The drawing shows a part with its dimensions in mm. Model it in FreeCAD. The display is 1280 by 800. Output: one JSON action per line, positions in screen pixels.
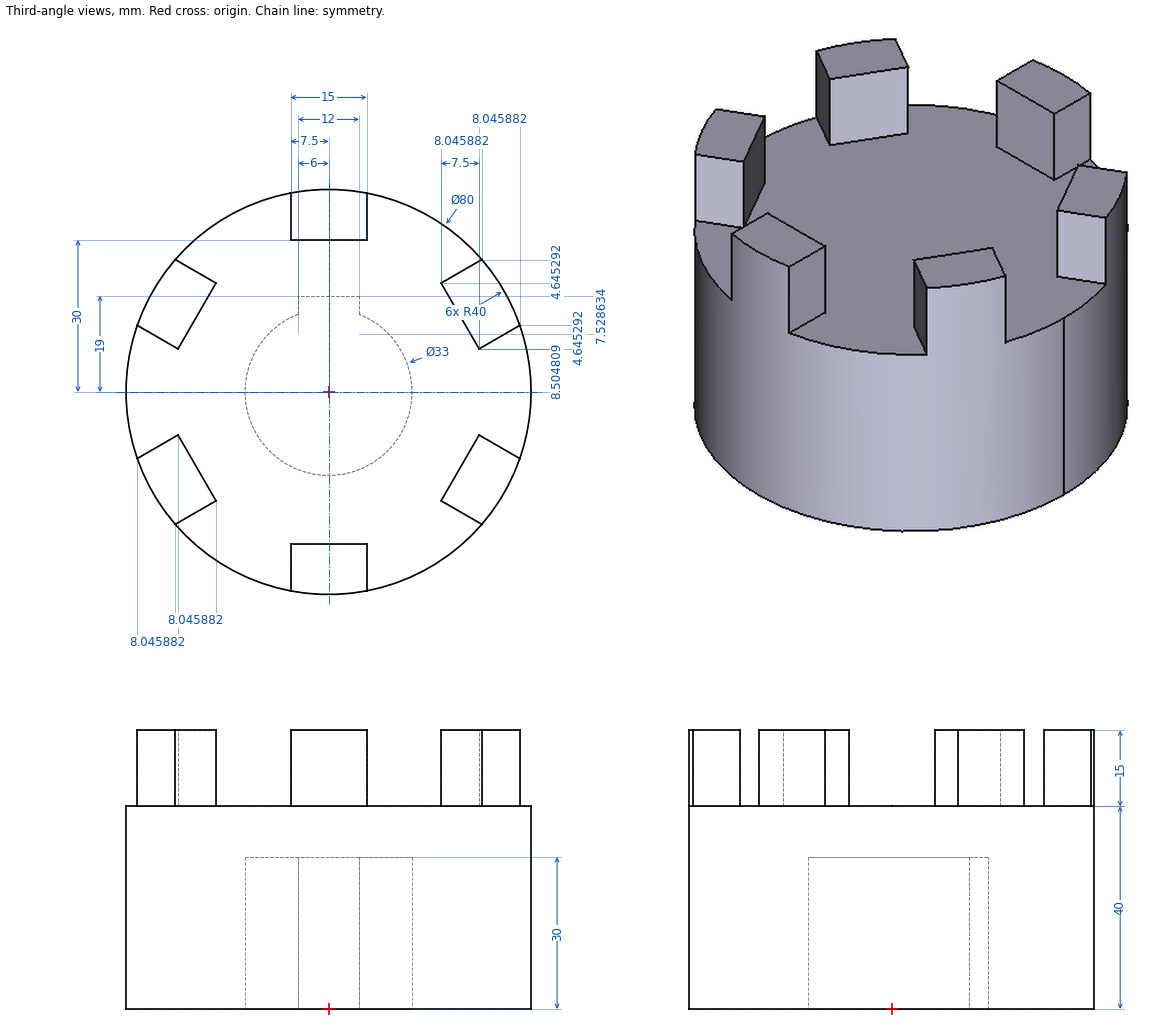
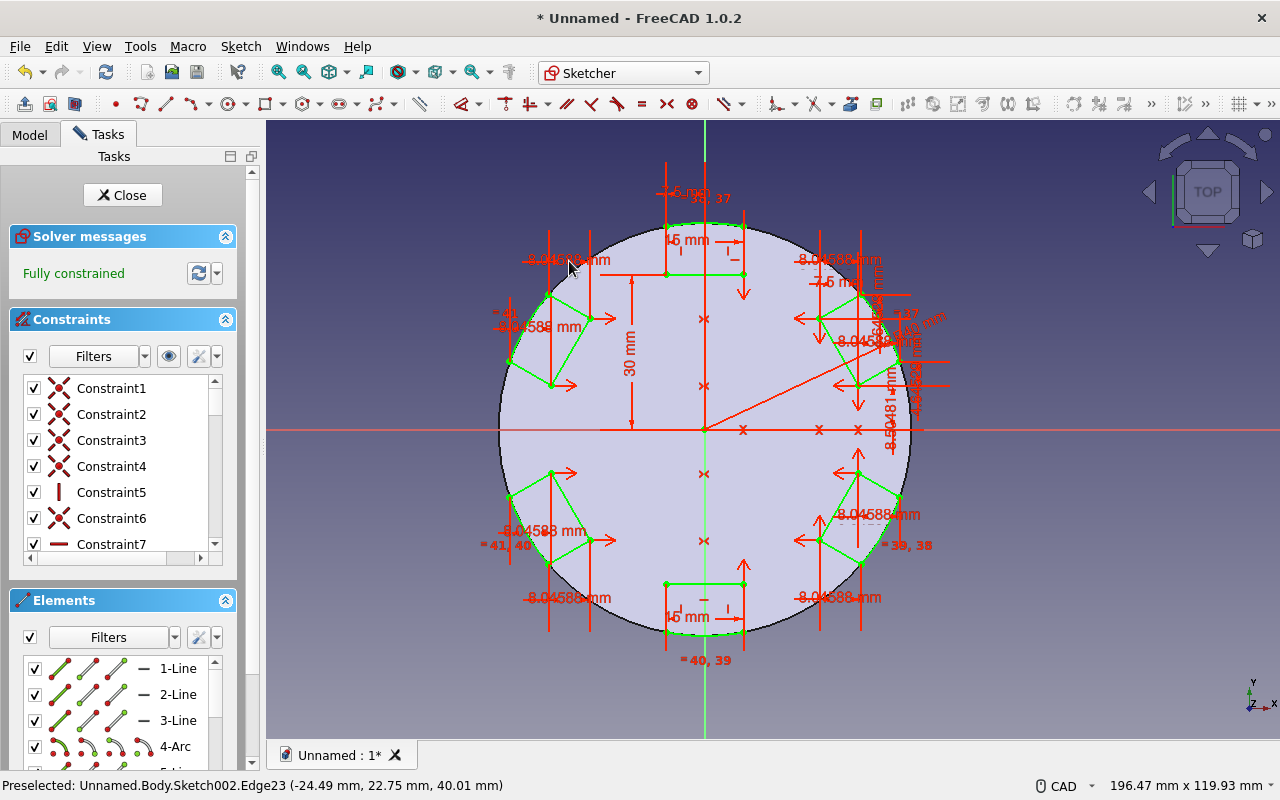
{"action": "left_click", "coordinate": [123, 195]}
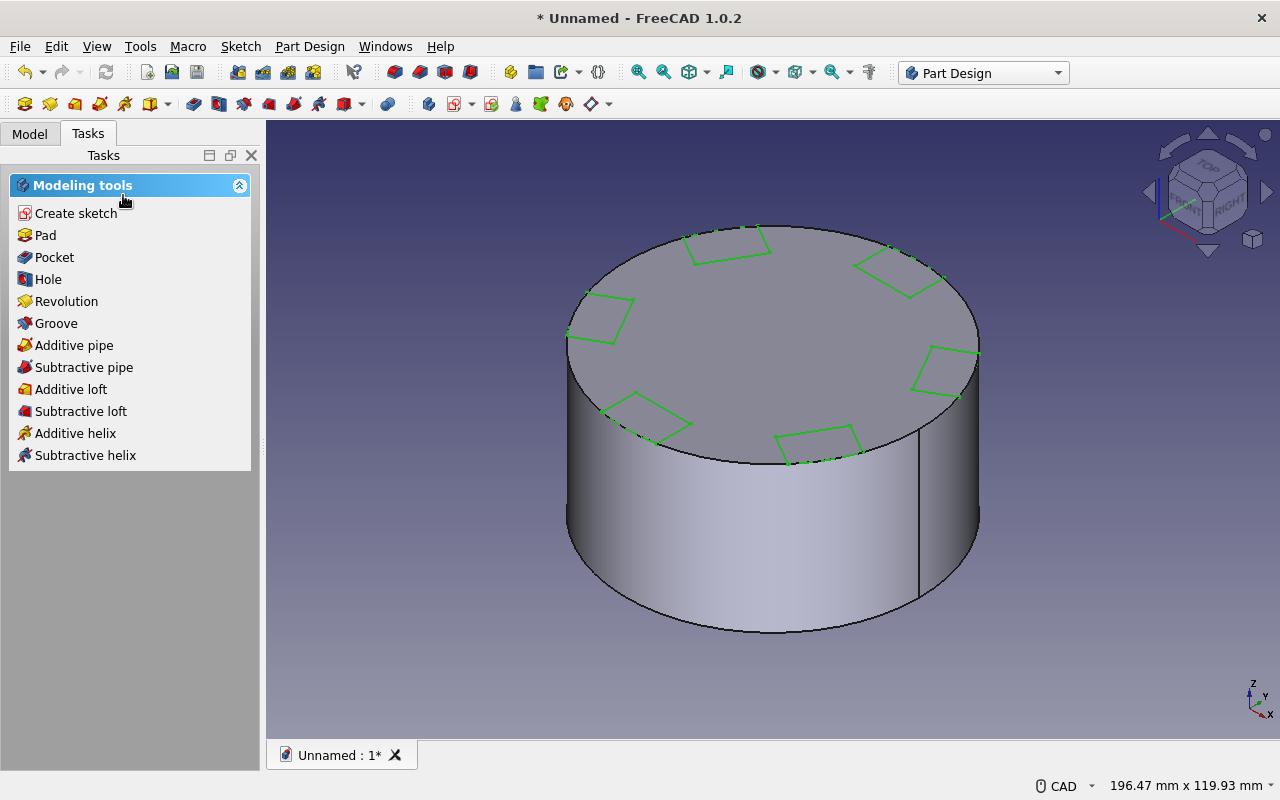
{"action": "left_click", "coordinate": [25, 104]}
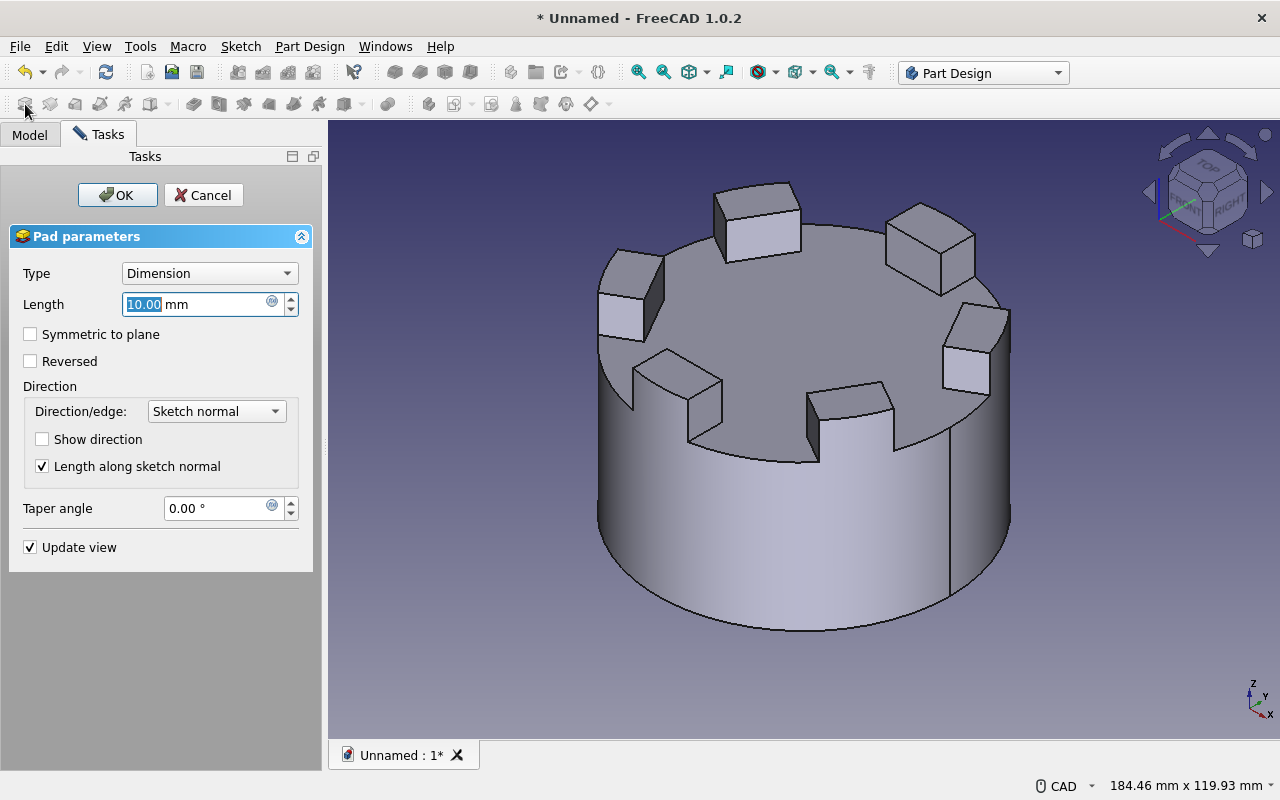
{"action": "type", "text": "15"}
{"action": "key", "text": "Tab"}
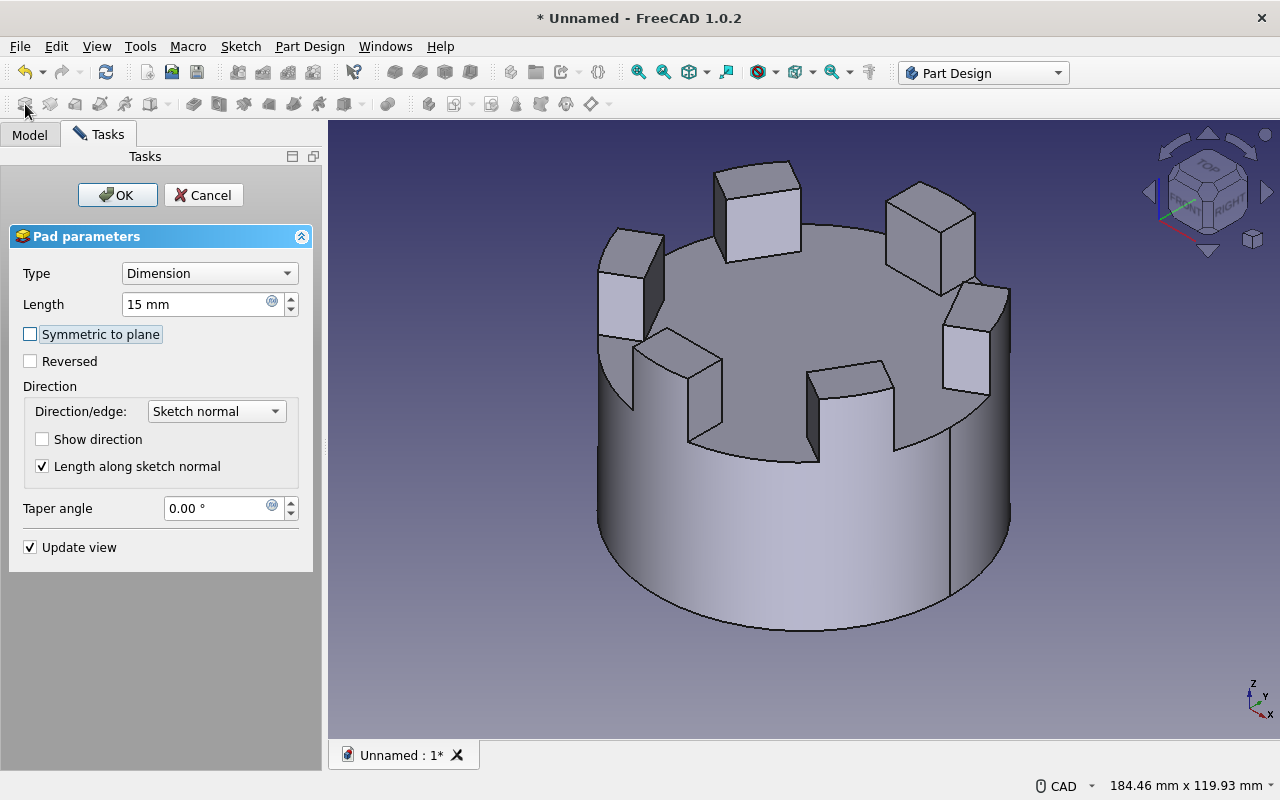
{"action": "left_click", "coordinate": [118, 195]}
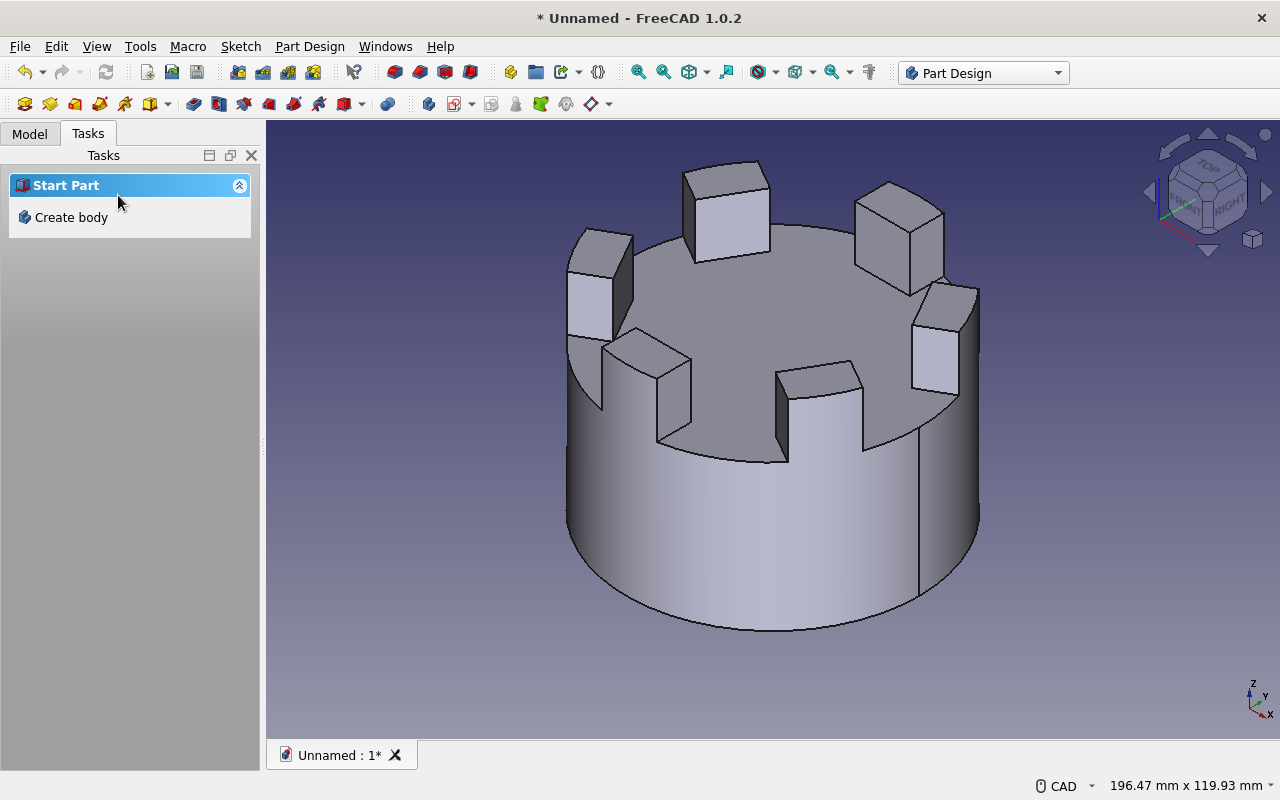
{"action": "key", "text": "v f"}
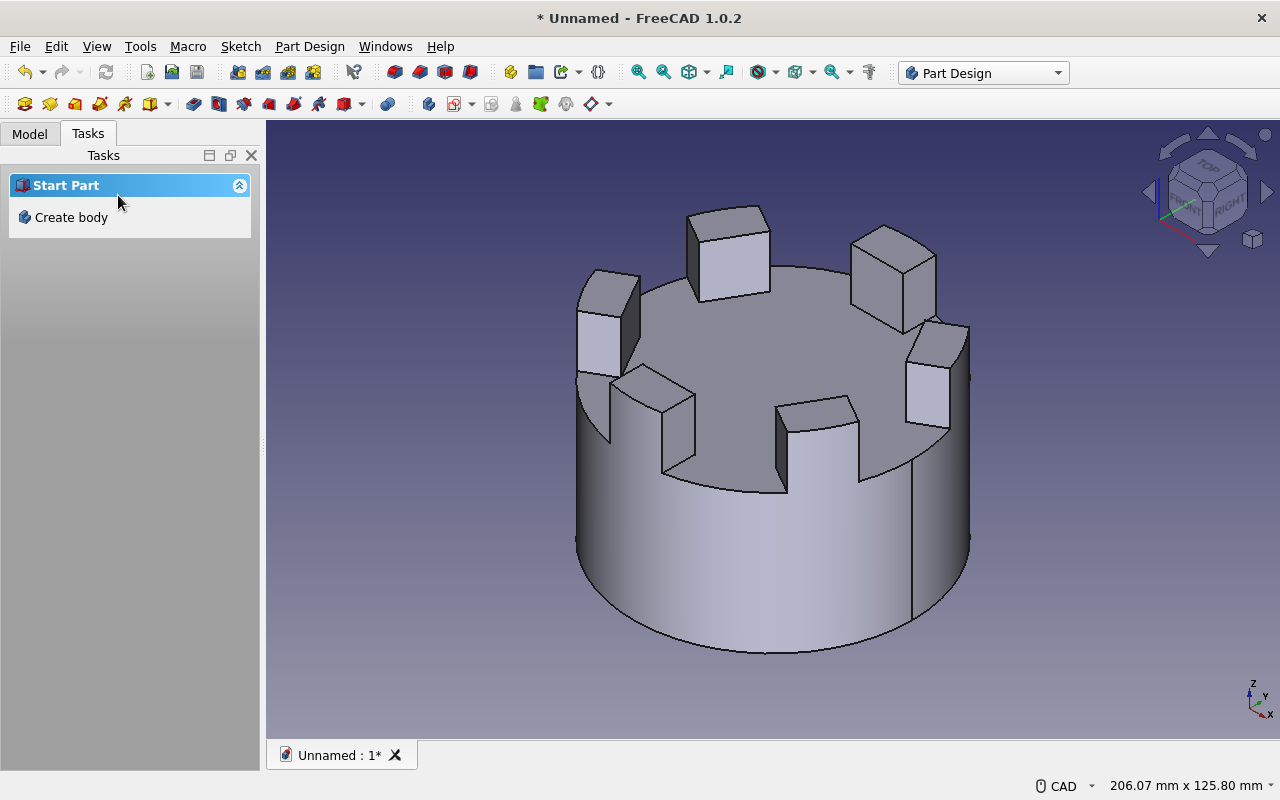
{"action": "key", "text": "5"}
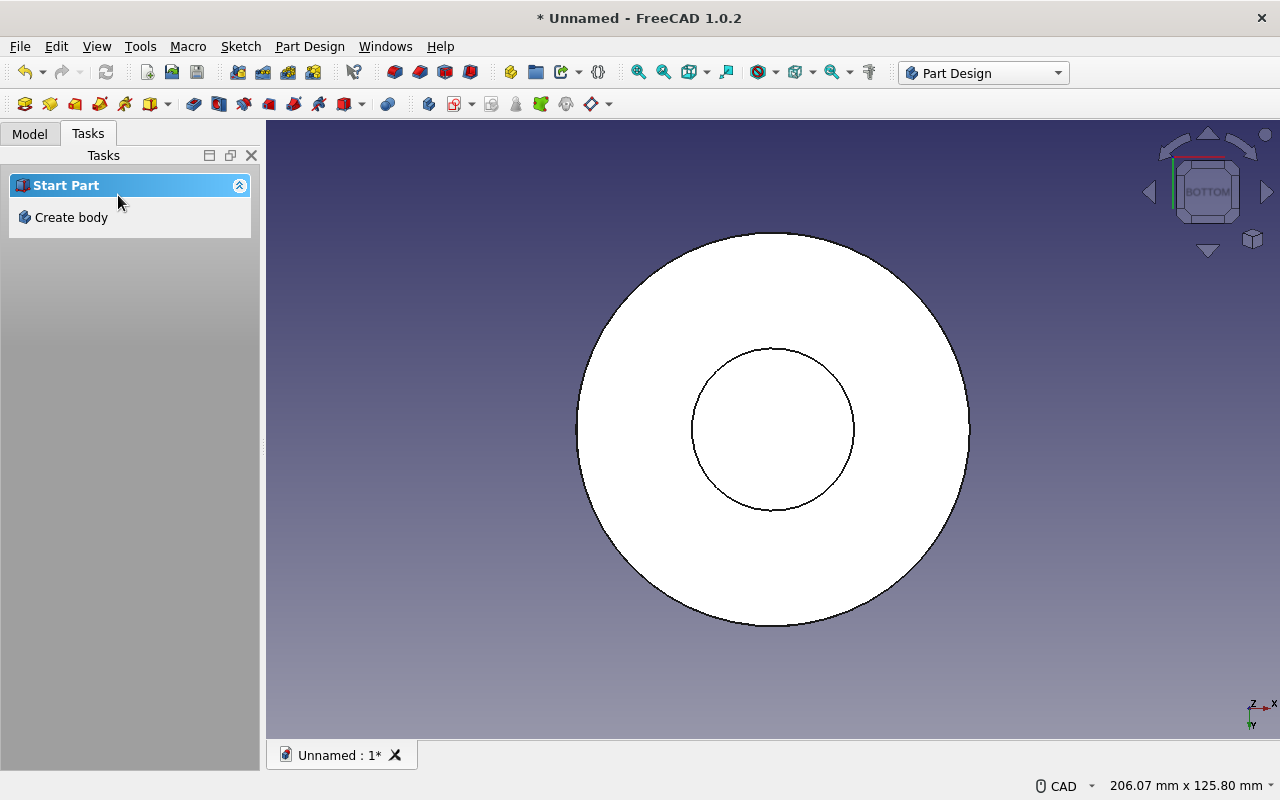
{"action": "left_click", "coordinate": [661, 485]}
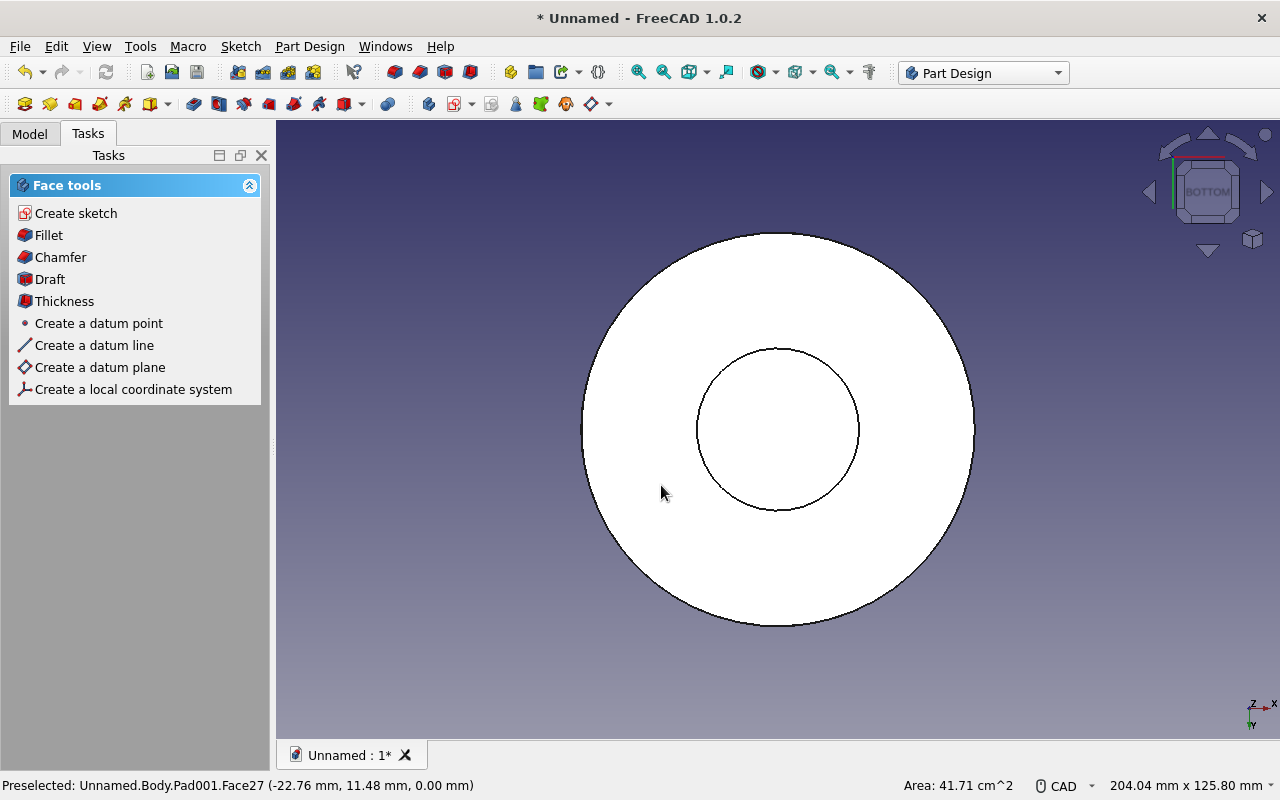
{"action": "left_click", "coordinate": [454, 104]}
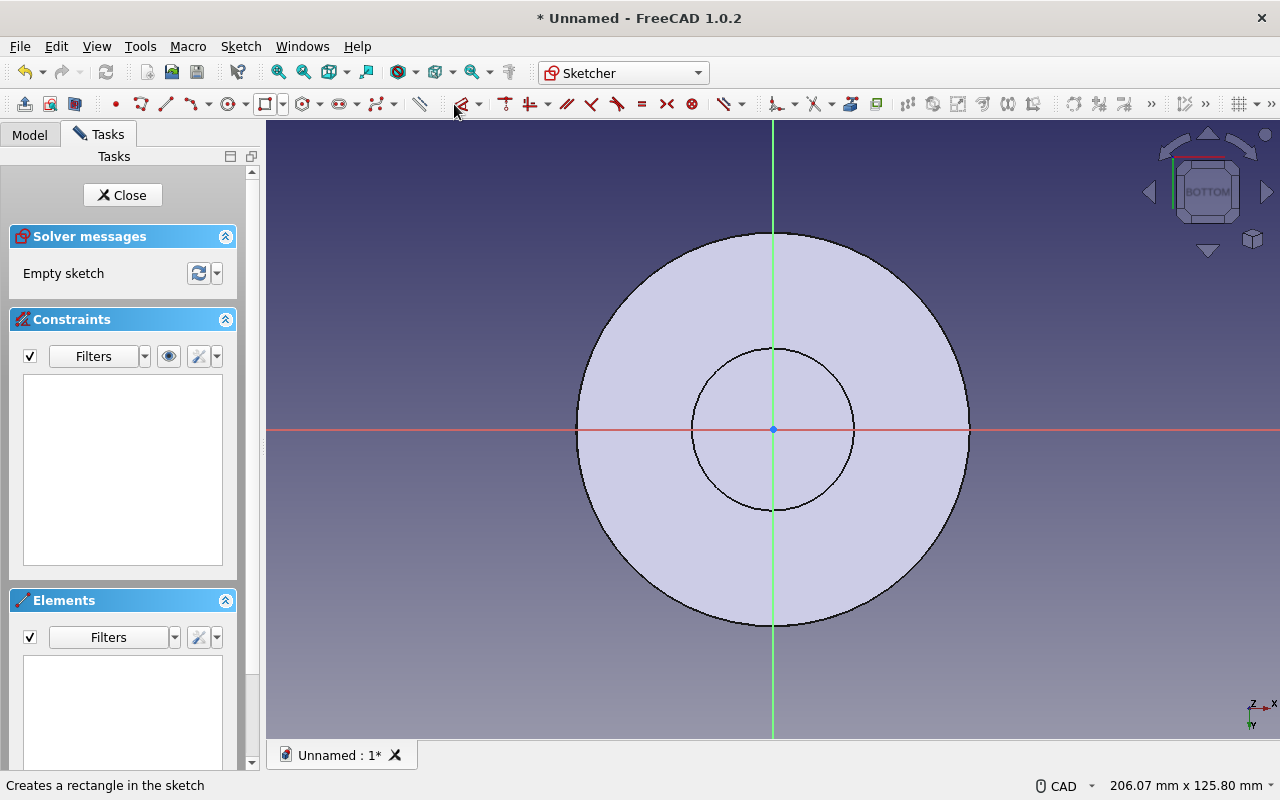
{"action": "scroll", "coordinate": [795, 492], "scroll_direction": "up", "scroll_amount": 7}